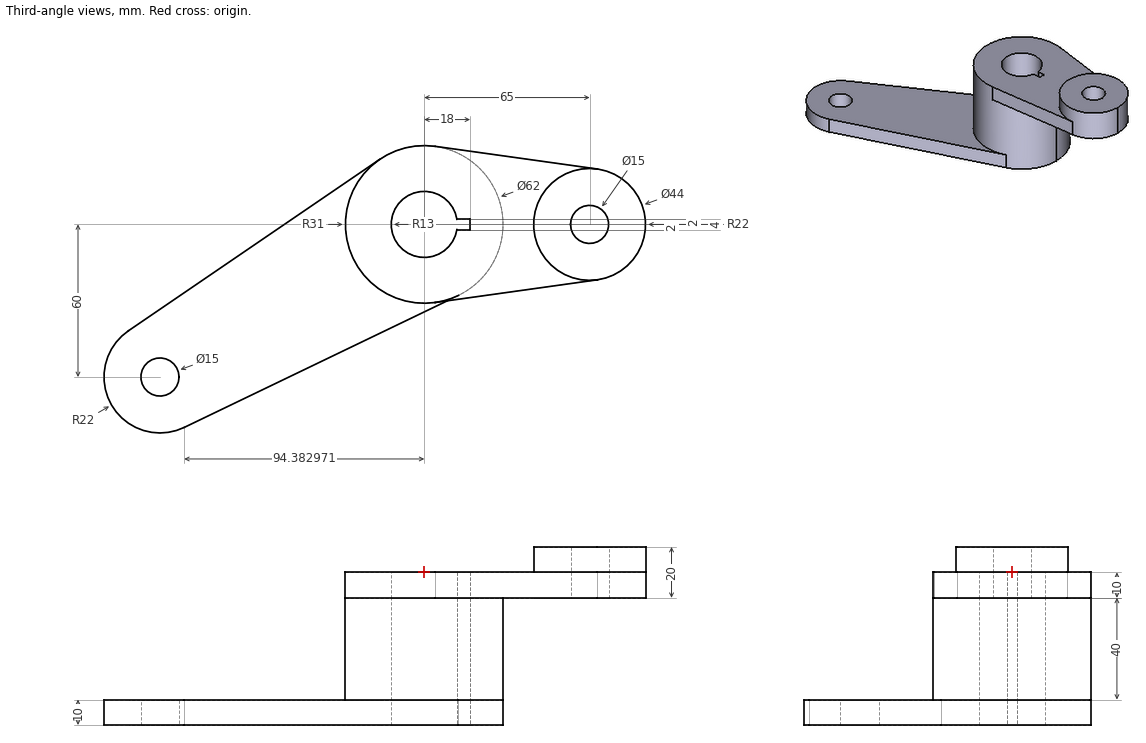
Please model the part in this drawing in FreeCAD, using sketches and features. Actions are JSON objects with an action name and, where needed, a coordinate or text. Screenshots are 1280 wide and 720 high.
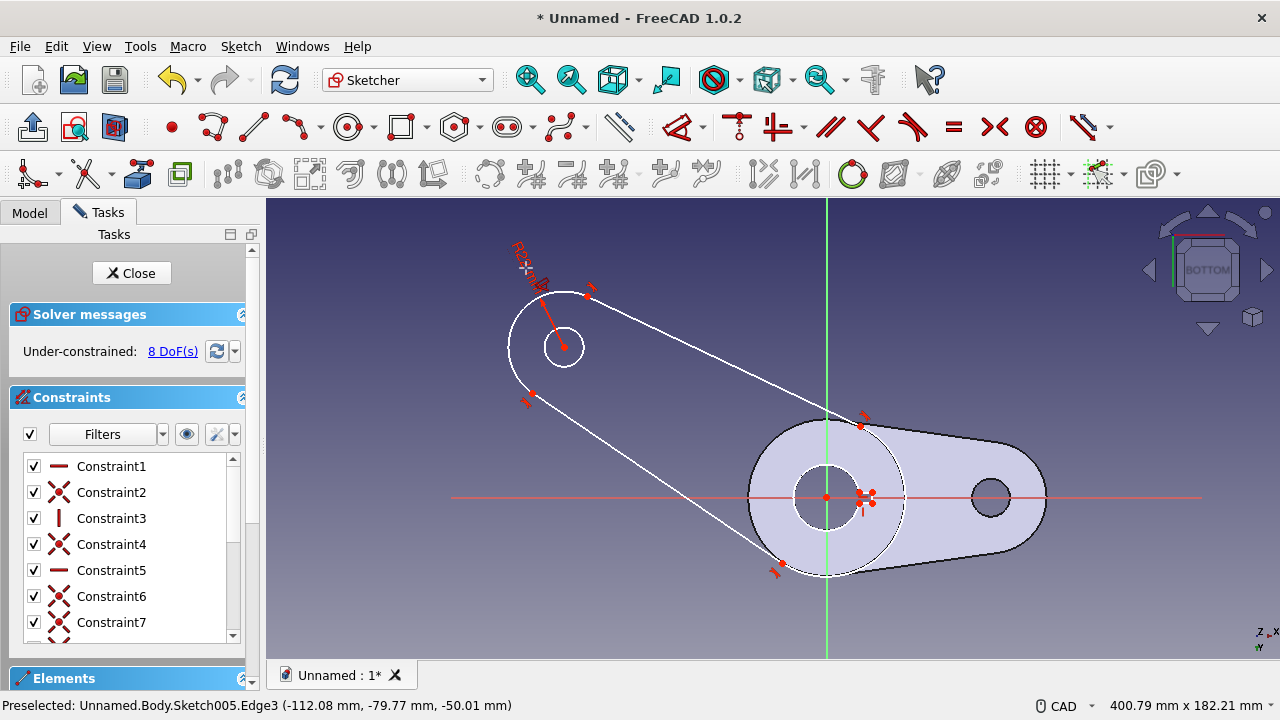
{"action": "left_click", "coordinate": [857, 571]}
{"action": "left_click", "coordinate": [869, 601]}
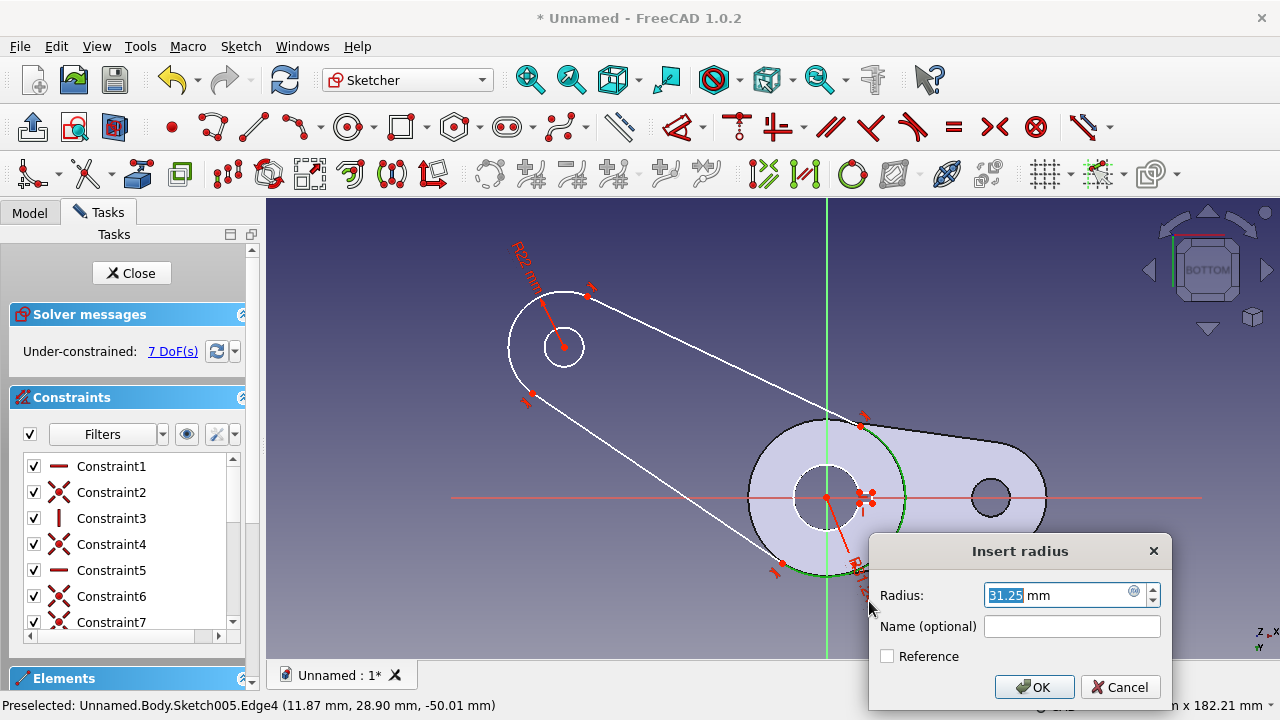
{"action": "type", "text": "31"}
{"action": "key", "text": "Return"}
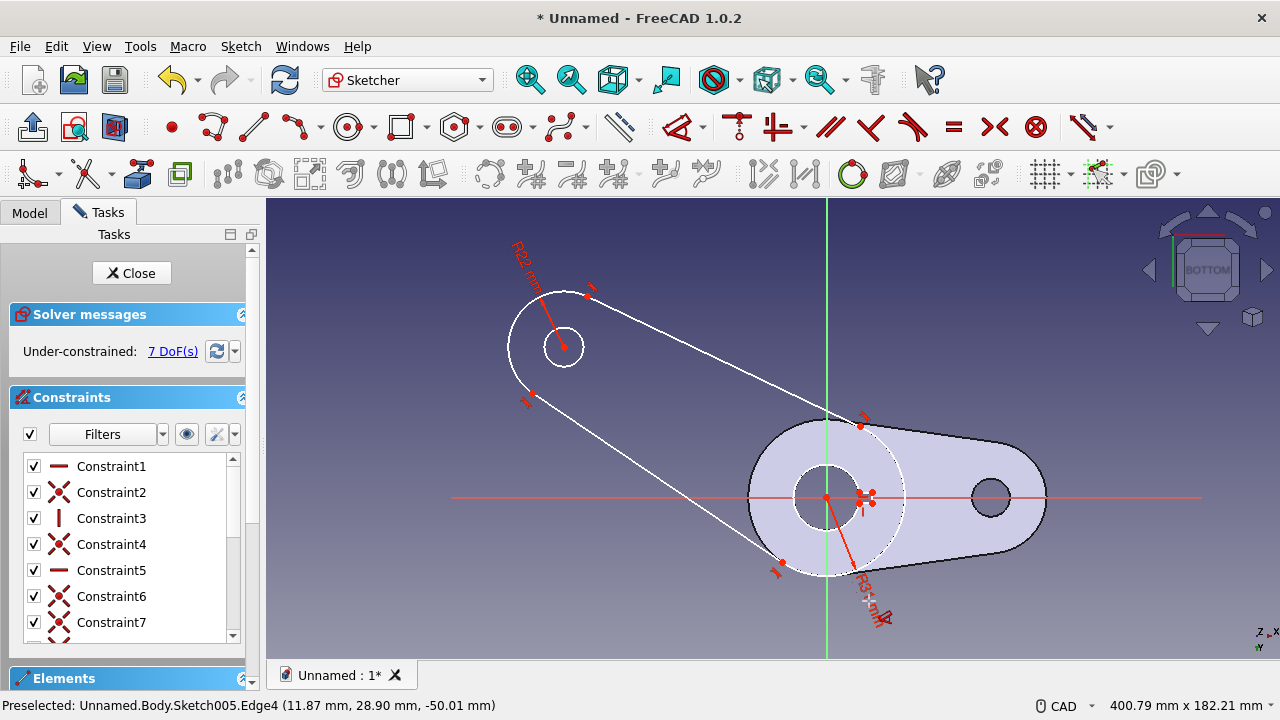
{"action": "left_click", "coordinate": [815, 467]}
{"action": "left_click", "coordinate": [804, 437]}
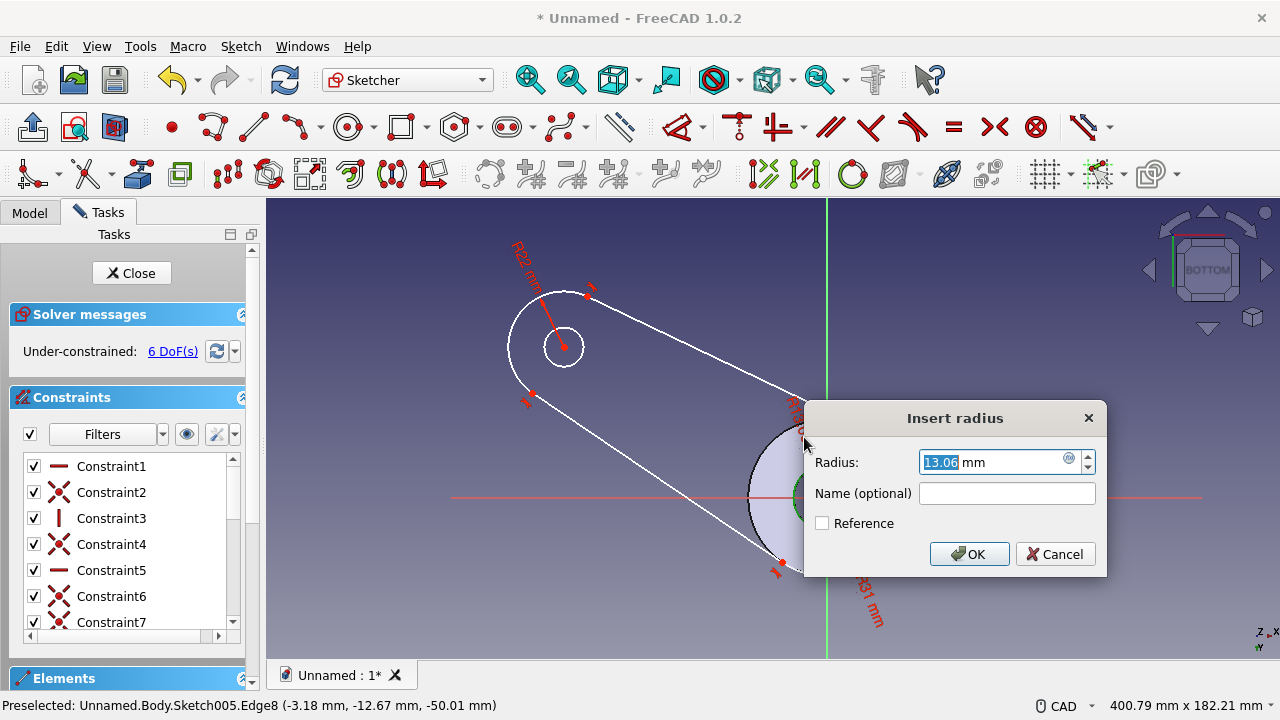
{"action": "type", "text": "13"}
{"action": "key", "text": "Return"}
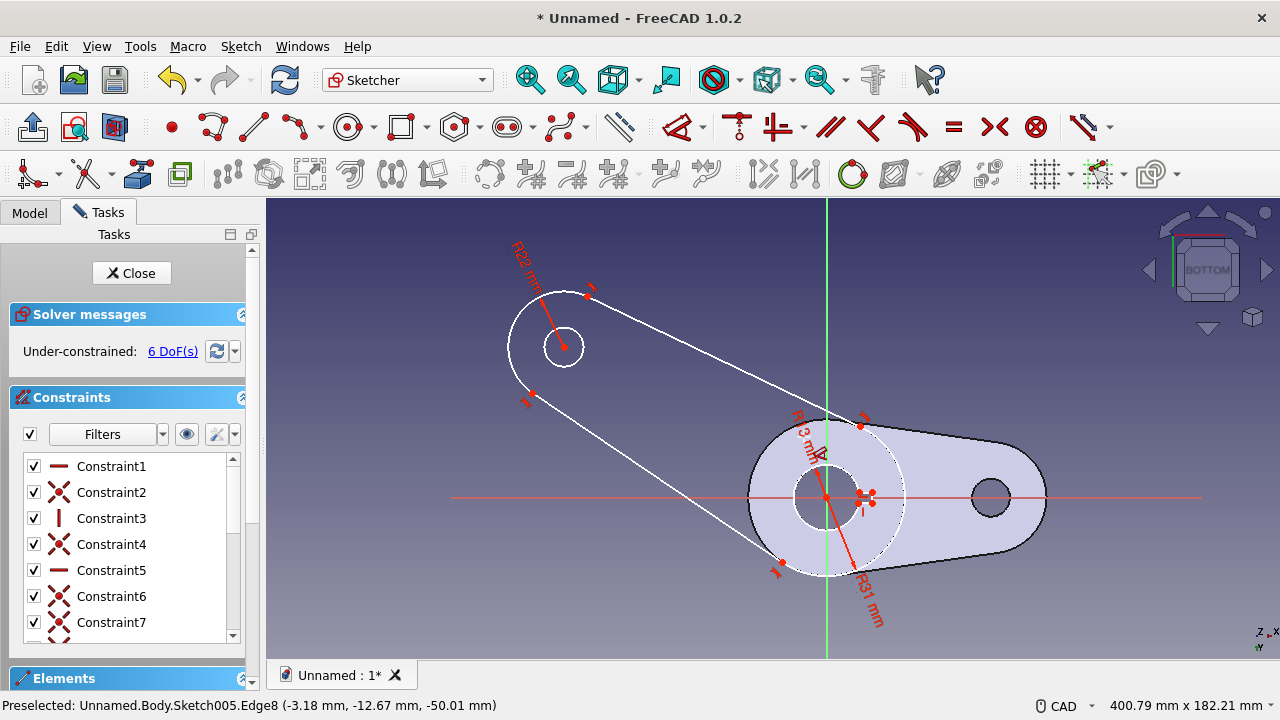
{"action": "left_click", "coordinate": [578, 333]}
{"action": "left_click", "coordinate": [614, 332]}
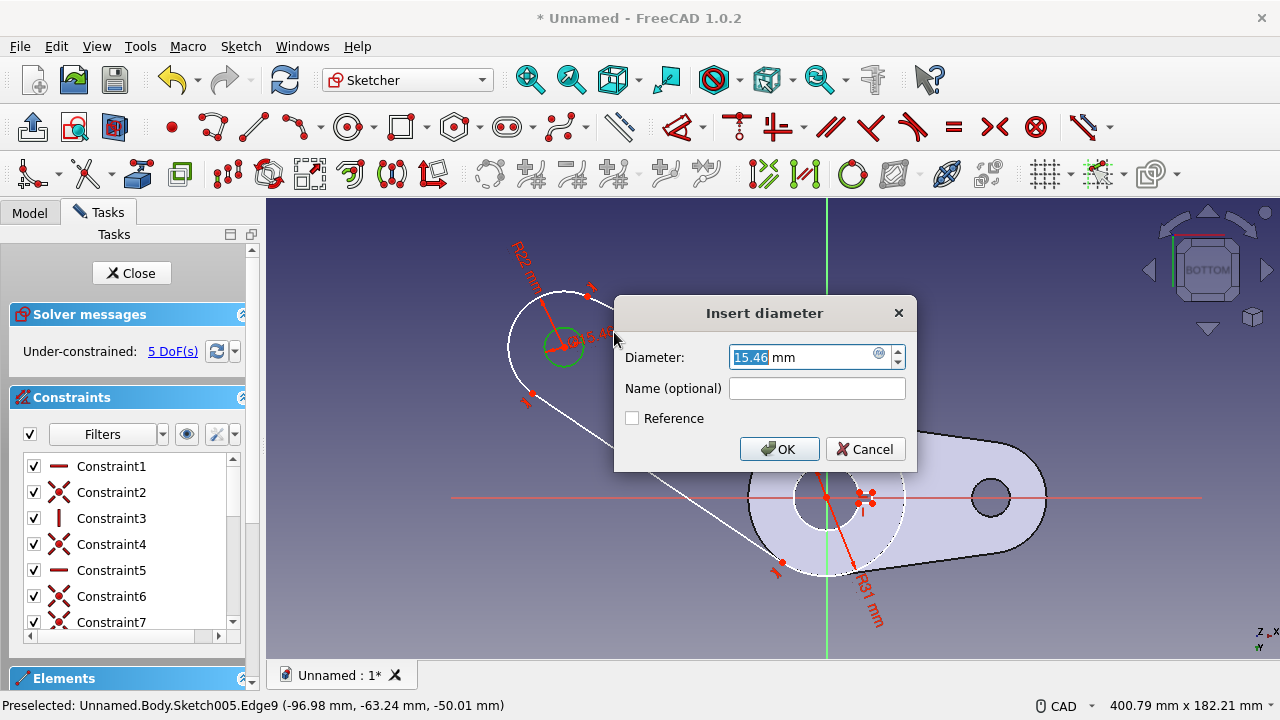
{"action": "type", "text": "15"}
{"action": "key", "text": "Return"}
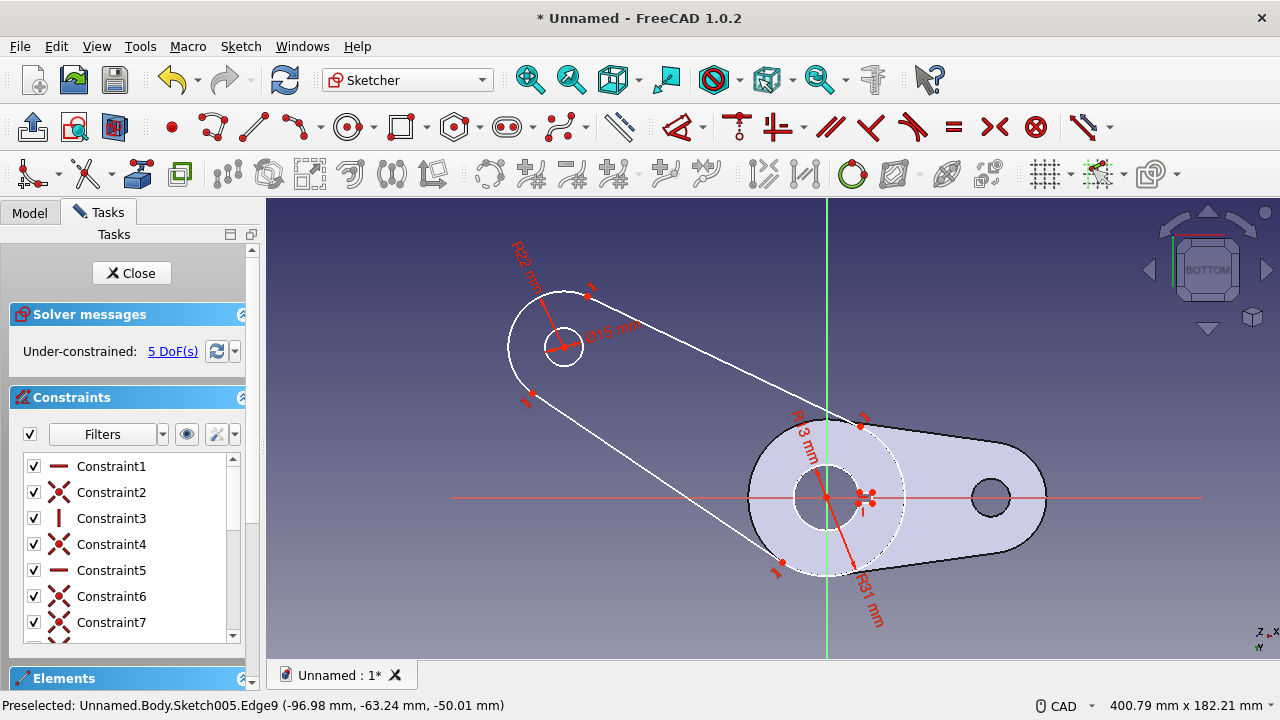
{"action": "scroll", "coordinate": [872, 498], "scroll_direction": "up", "scroll_amount": 7}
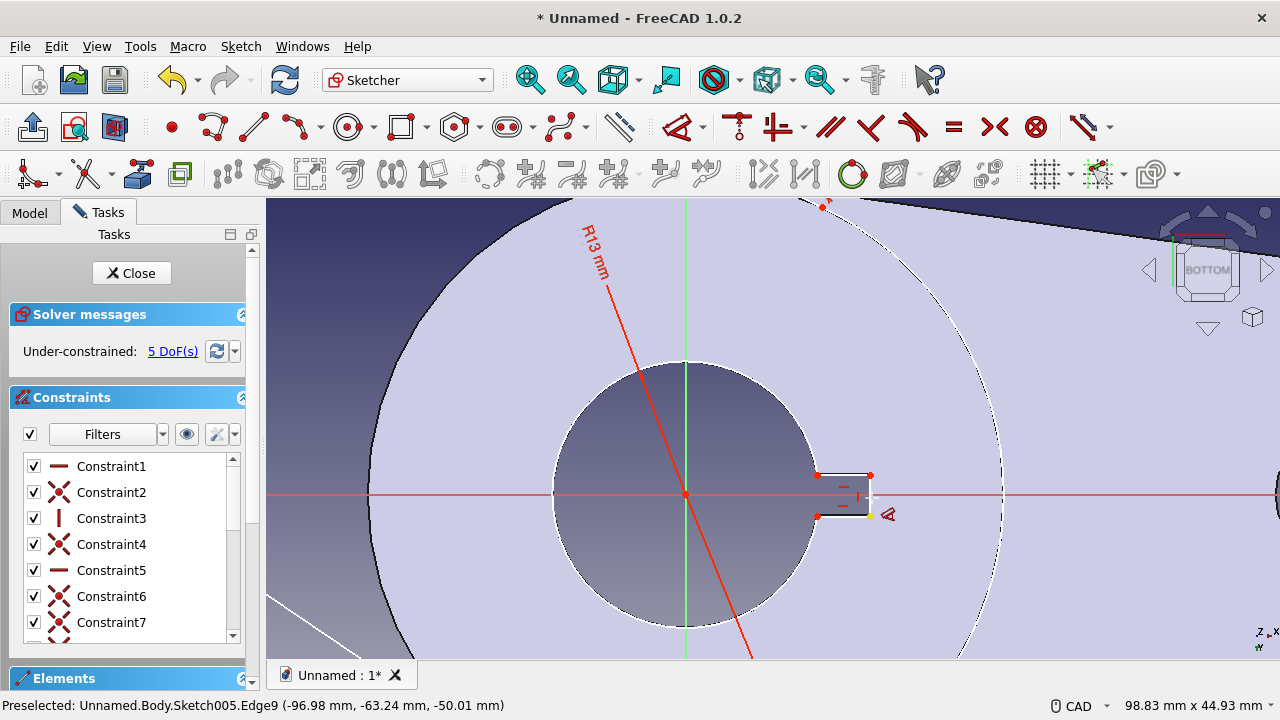
{"action": "left_click", "coordinate": [870, 496]}
{"action": "left_click", "coordinate": [904, 482]}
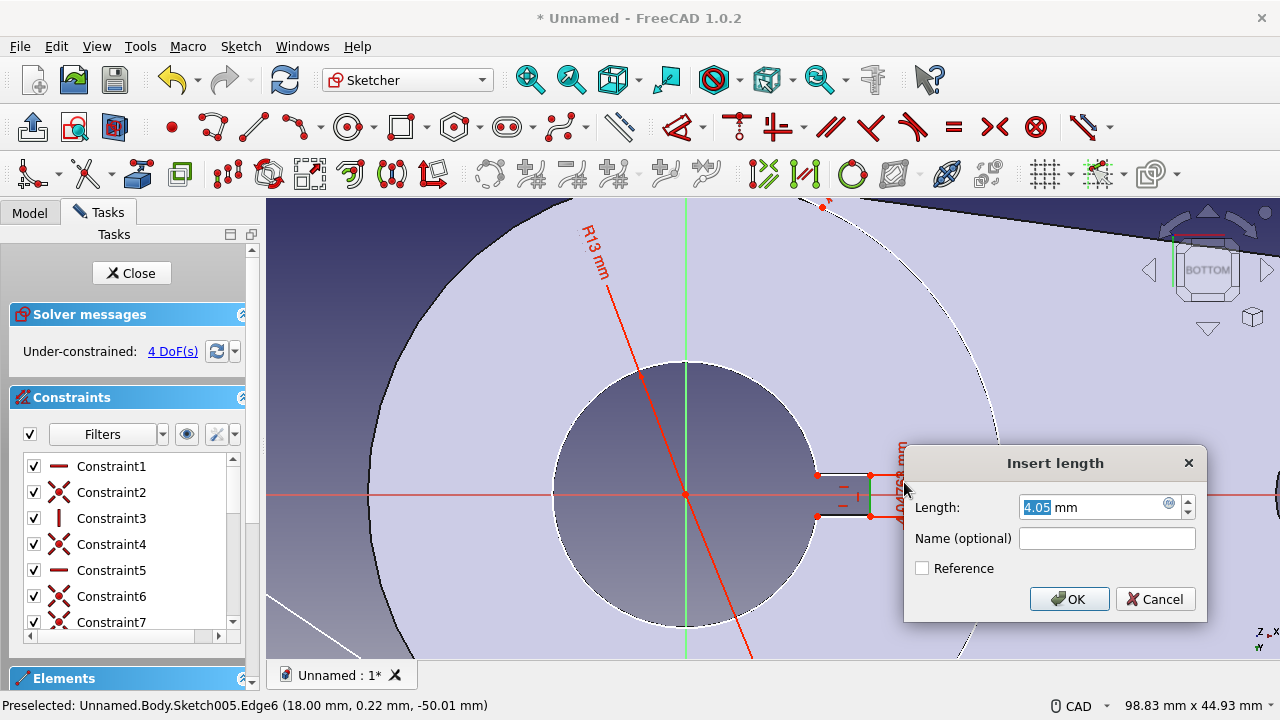
{"action": "type", "text": "4"}
{"action": "key", "text": "Return"}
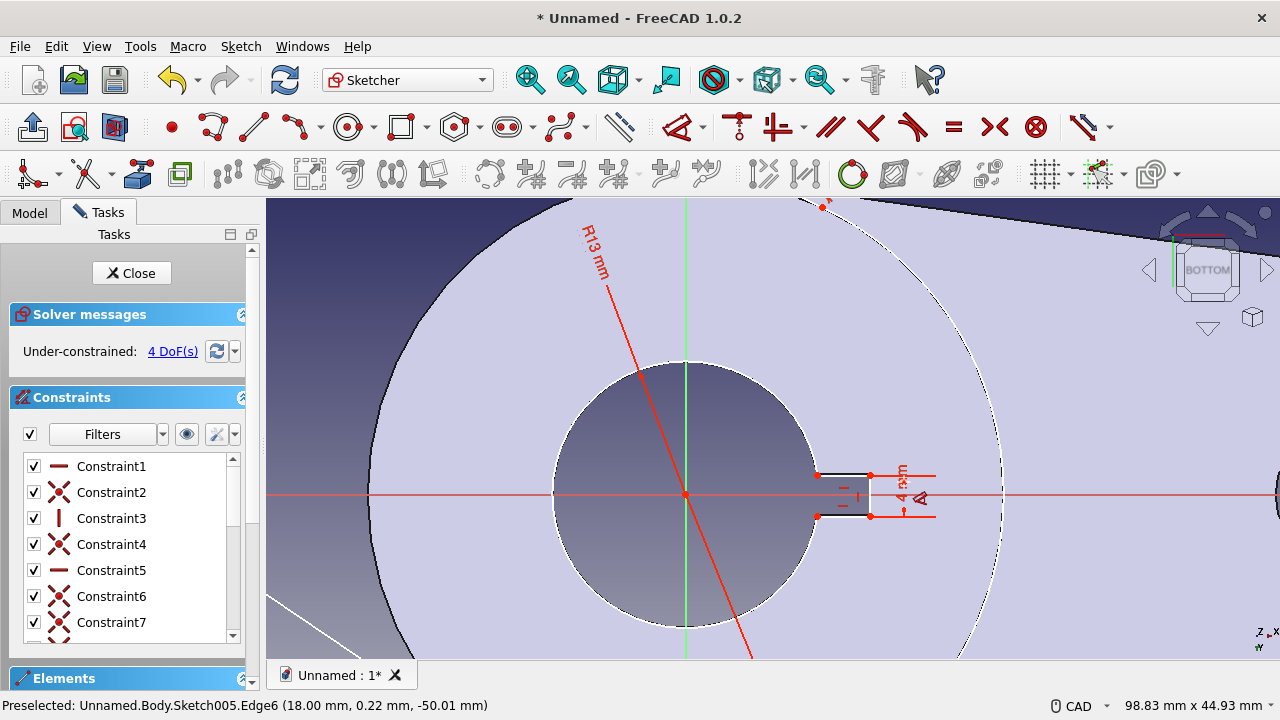
{"action": "scroll", "coordinate": [817, 517], "scroll_direction": "up", "scroll_amount": 4}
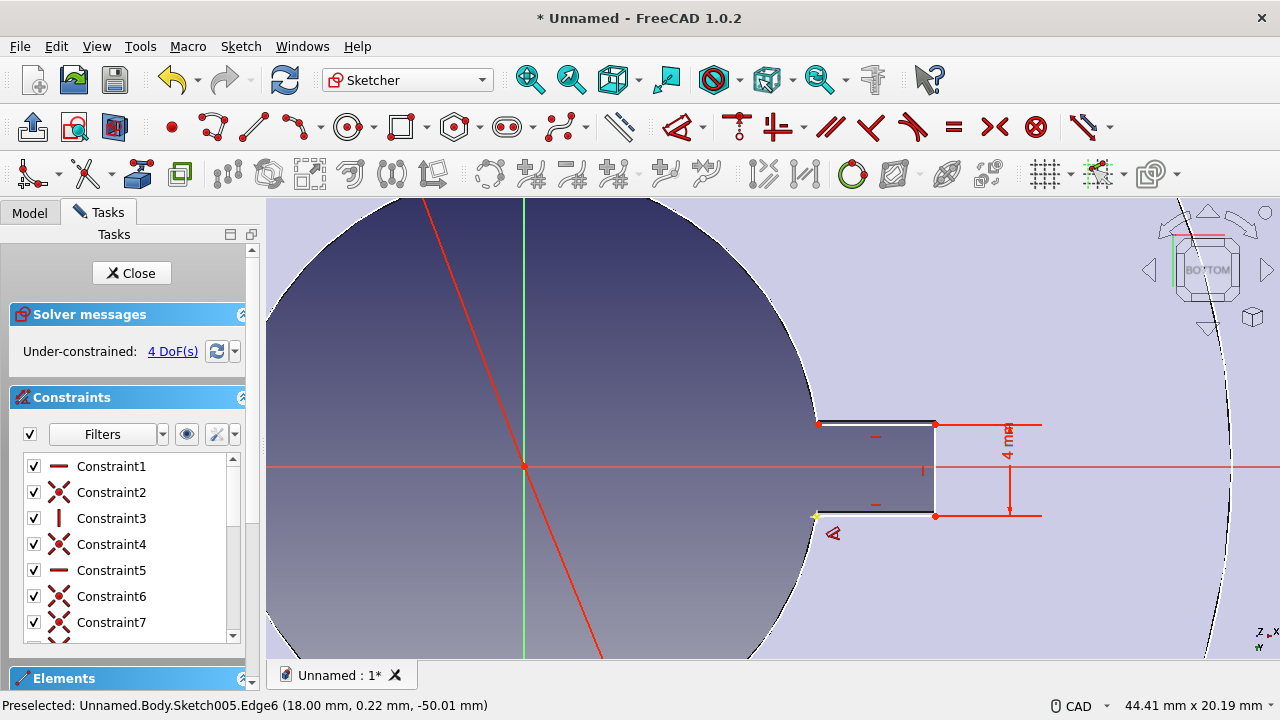
{"action": "left_click", "coordinate": [817, 516]}
{"action": "left_click", "coordinate": [851, 491]}